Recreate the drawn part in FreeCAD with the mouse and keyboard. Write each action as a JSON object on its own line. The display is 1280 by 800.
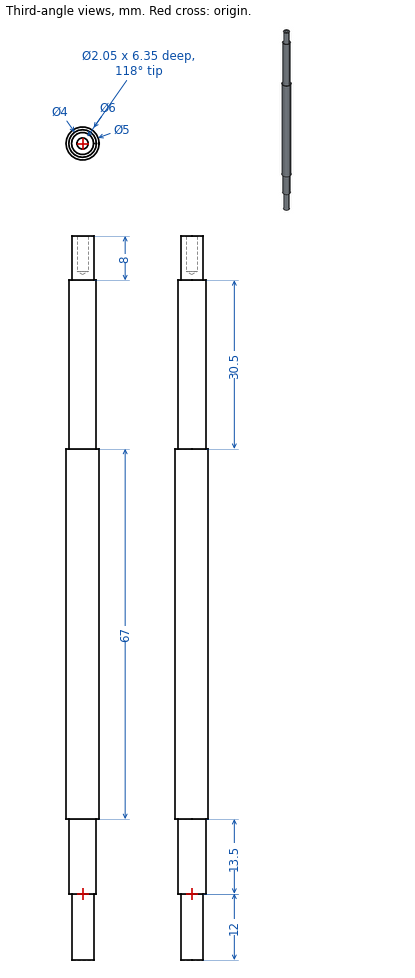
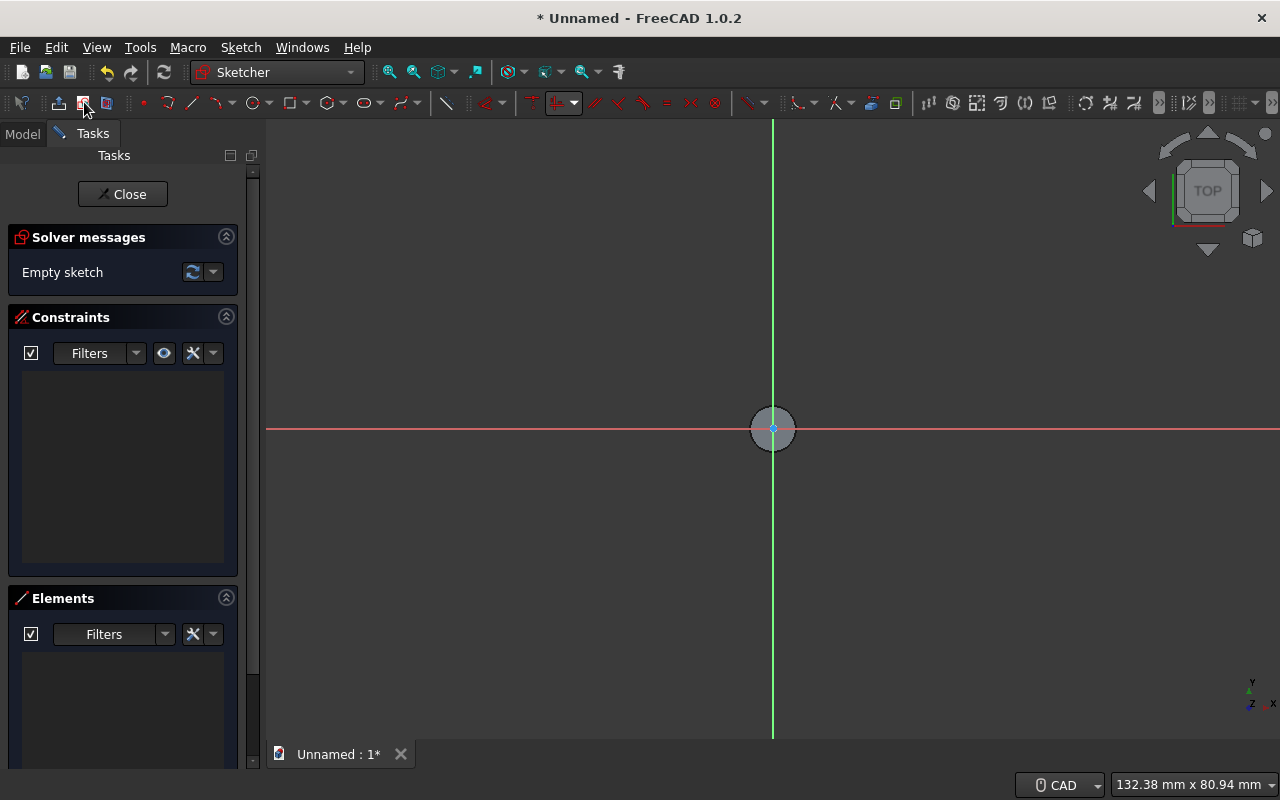
{"action": "scroll", "coordinate": [780, 429], "scroll_direction": "up", "scroll_amount": 12}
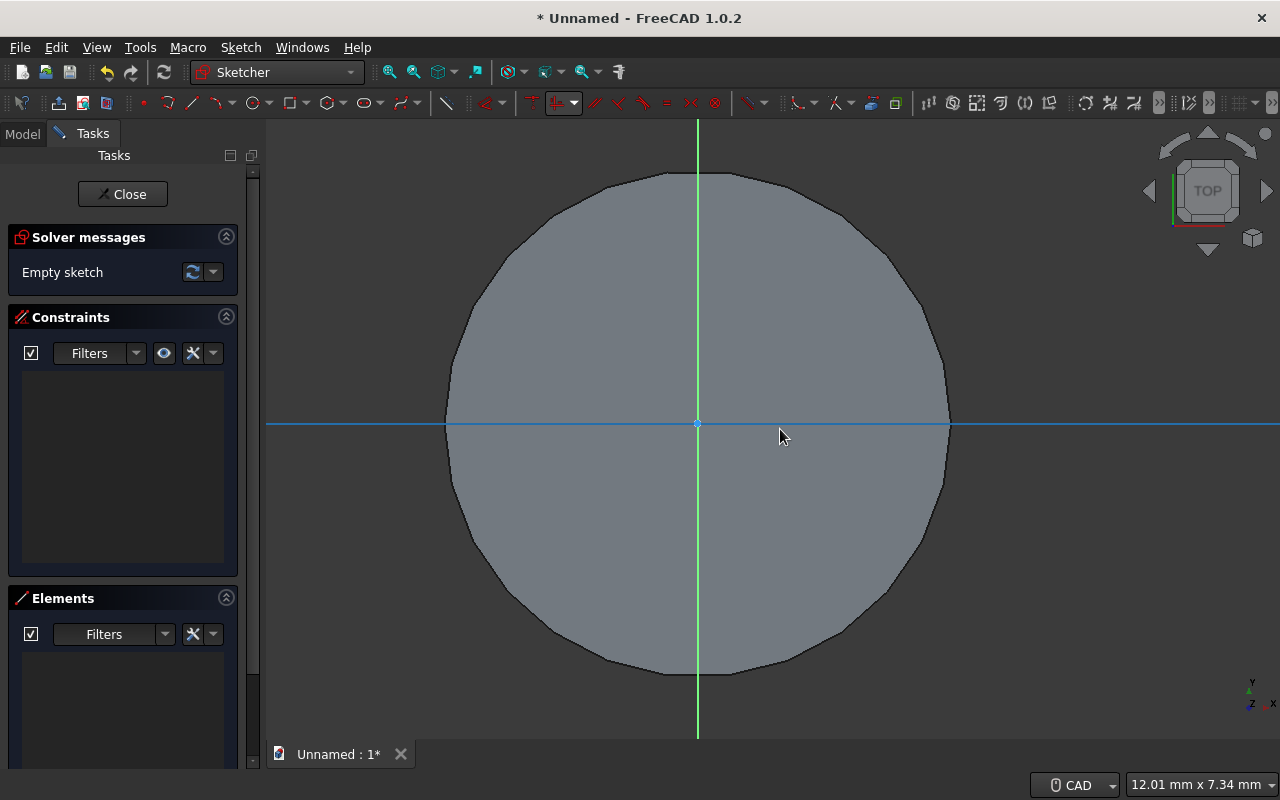
{"action": "left_click", "coordinate": [254, 104]}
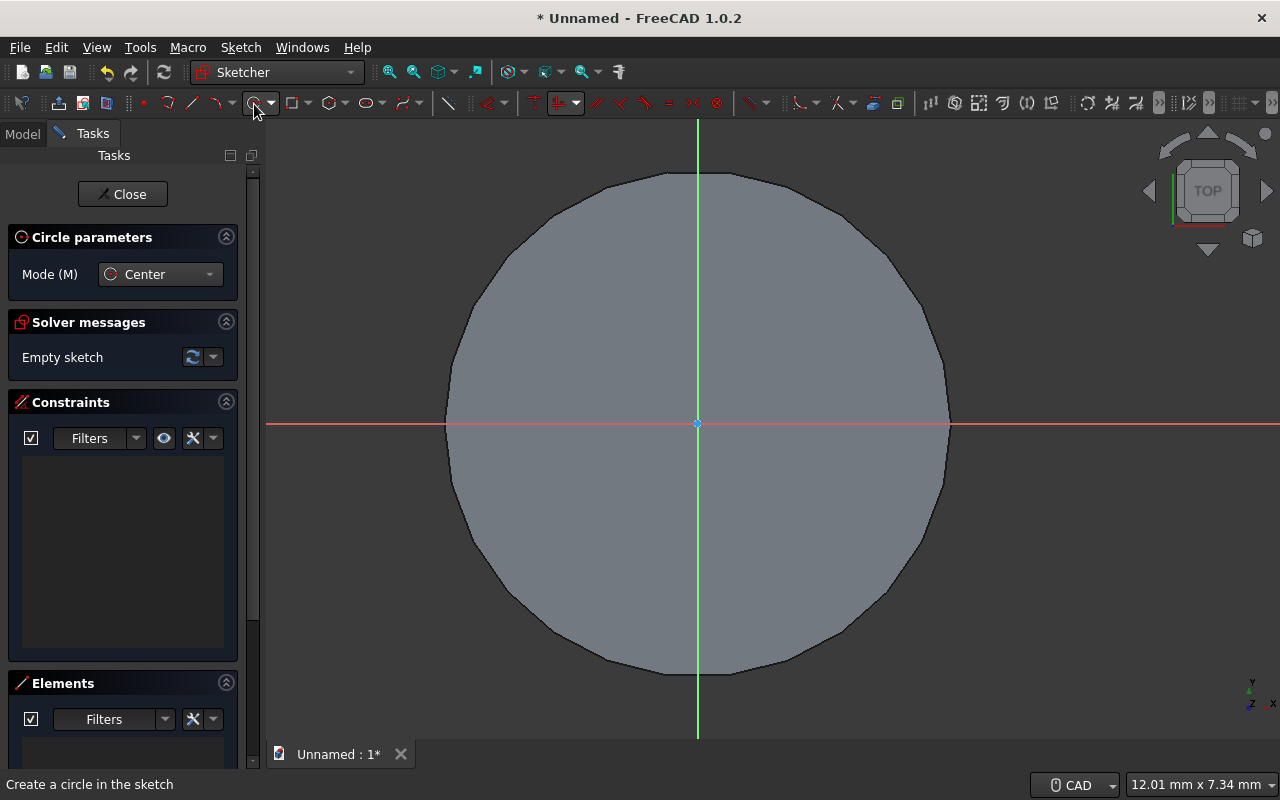
{"action": "left_click", "coordinate": [698, 424]}
{"action": "left_click", "coordinate": [847, 275]}
{"action": "key", "text": "Escape"}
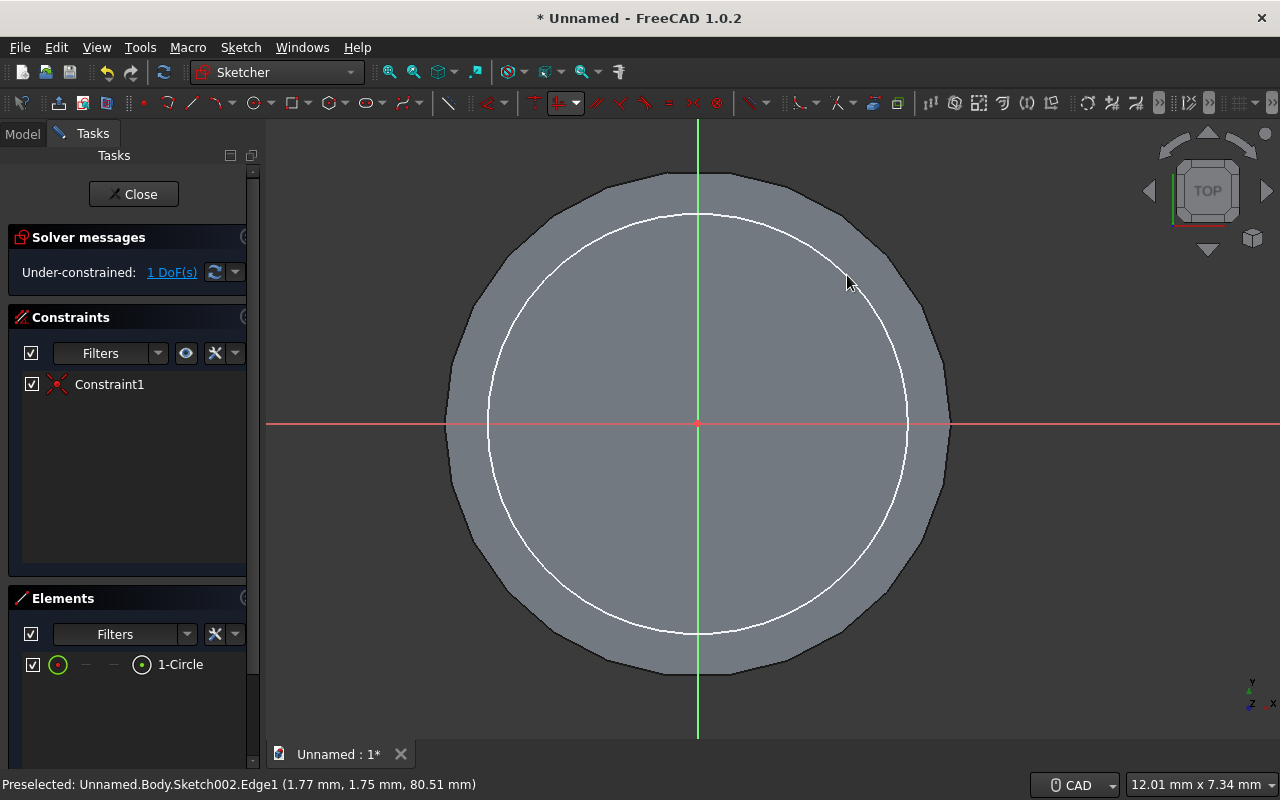
{"action": "left_click", "coordinate": [488, 104]}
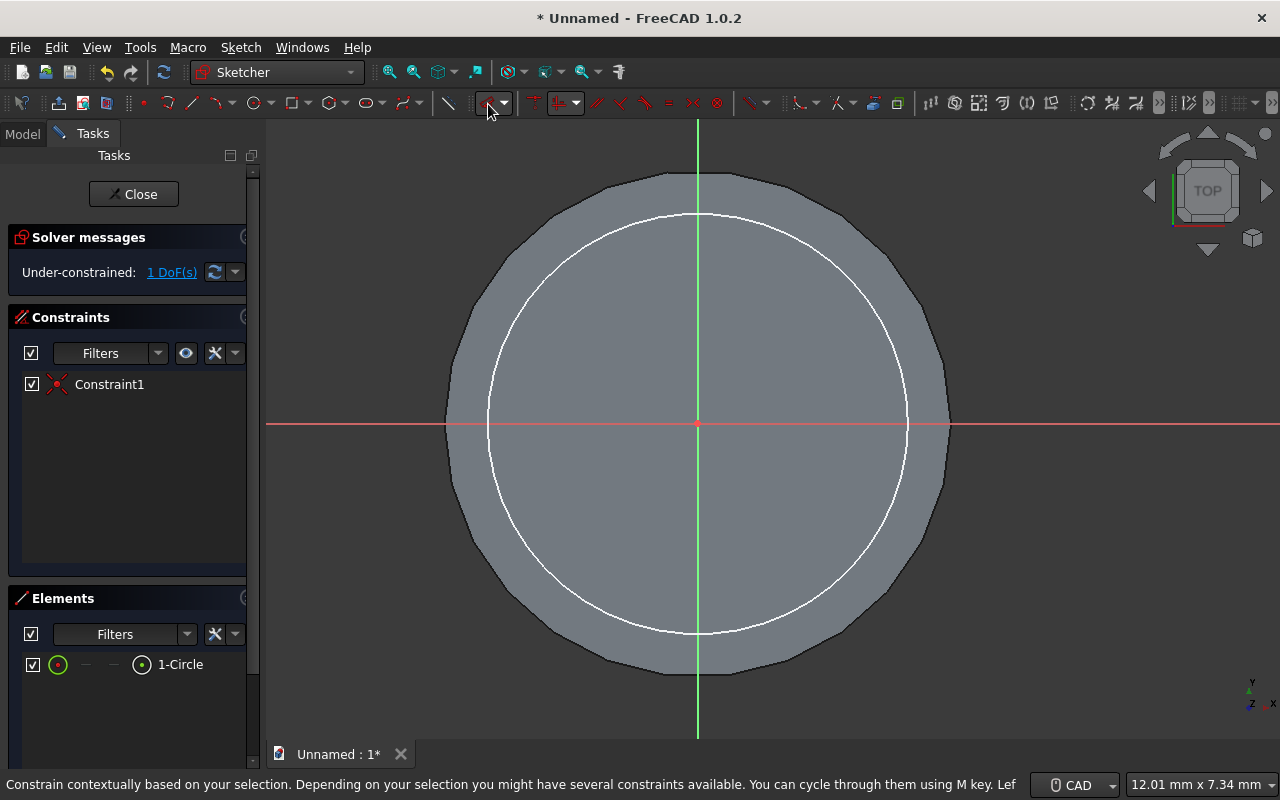
{"action": "left_click", "coordinate": [846, 275]}
{"action": "left_click", "coordinate": [869, 252]}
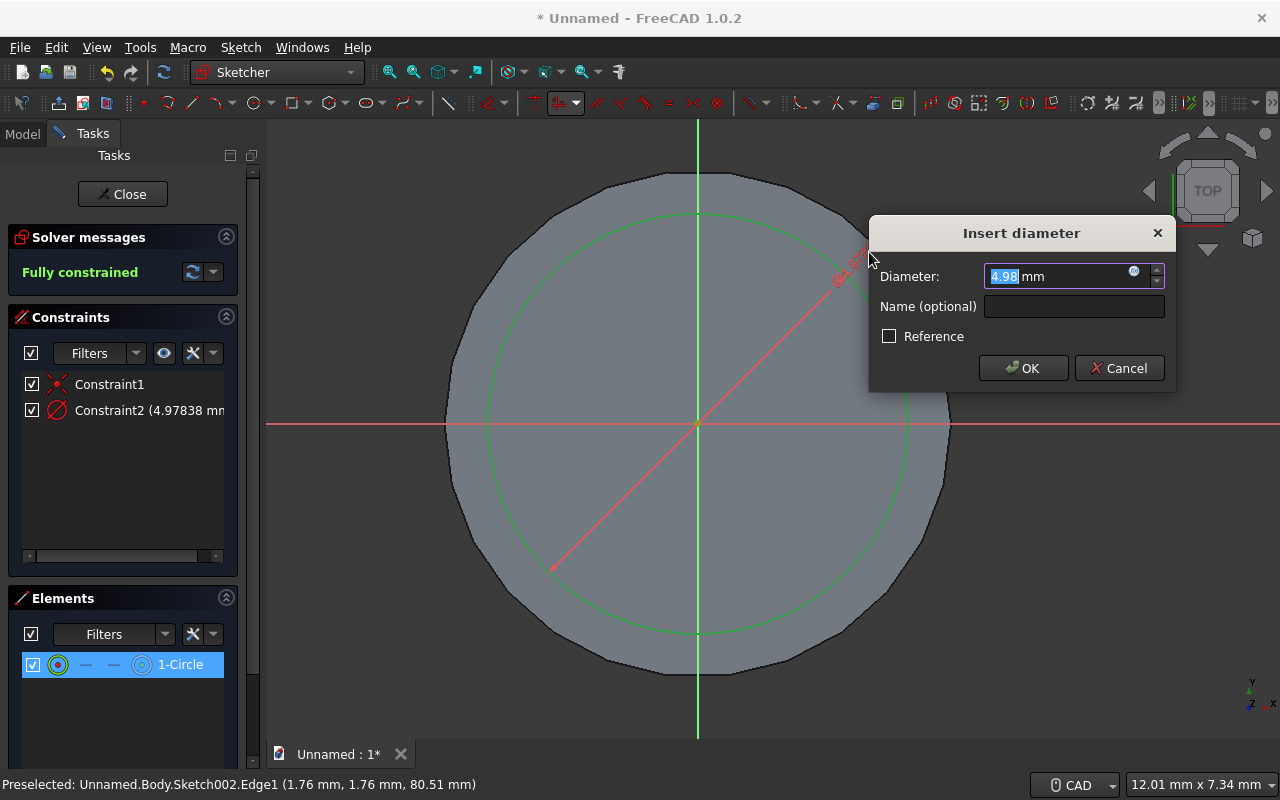
{"action": "type", "text": "5"}
{"action": "key", "text": "Return"}
{"action": "key", "text": "Escape"}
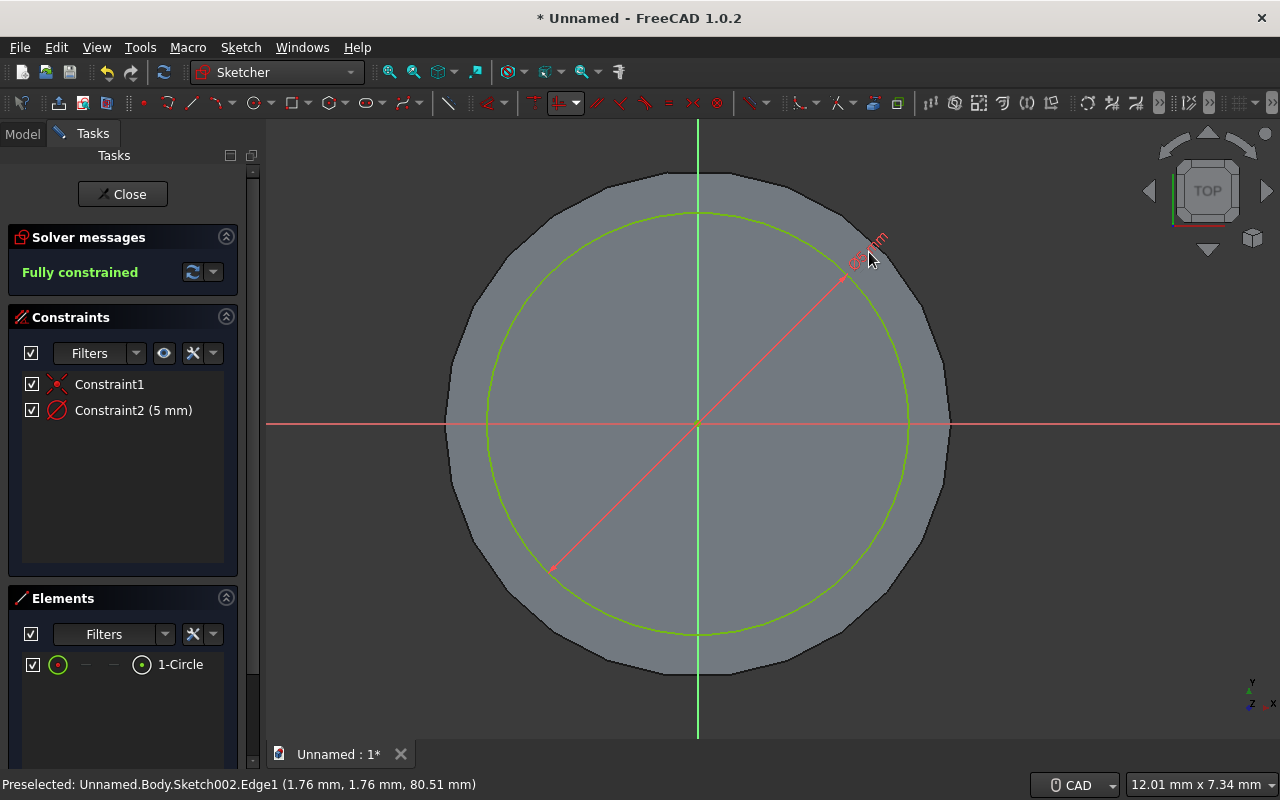
{"action": "left_click", "coordinate": [123, 194]}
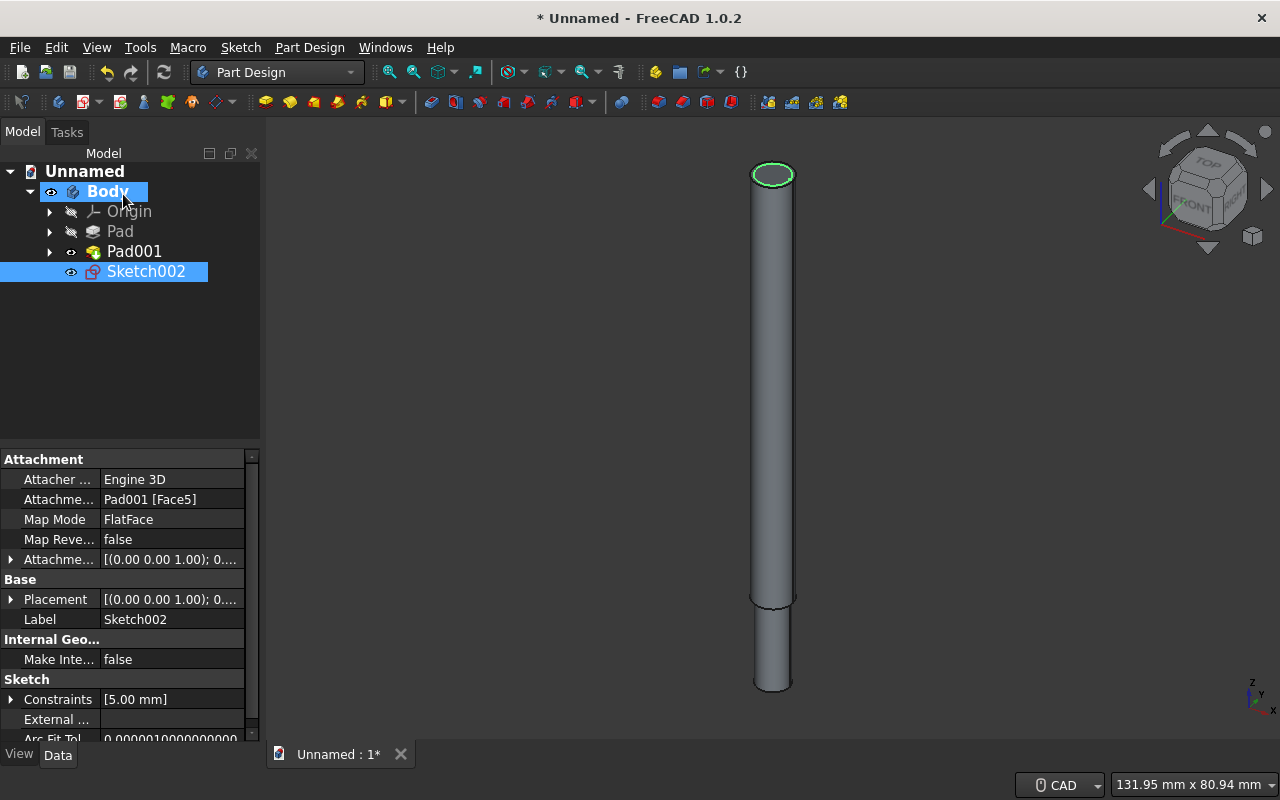
{"action": "left_click", "coordinate": [266, 102]}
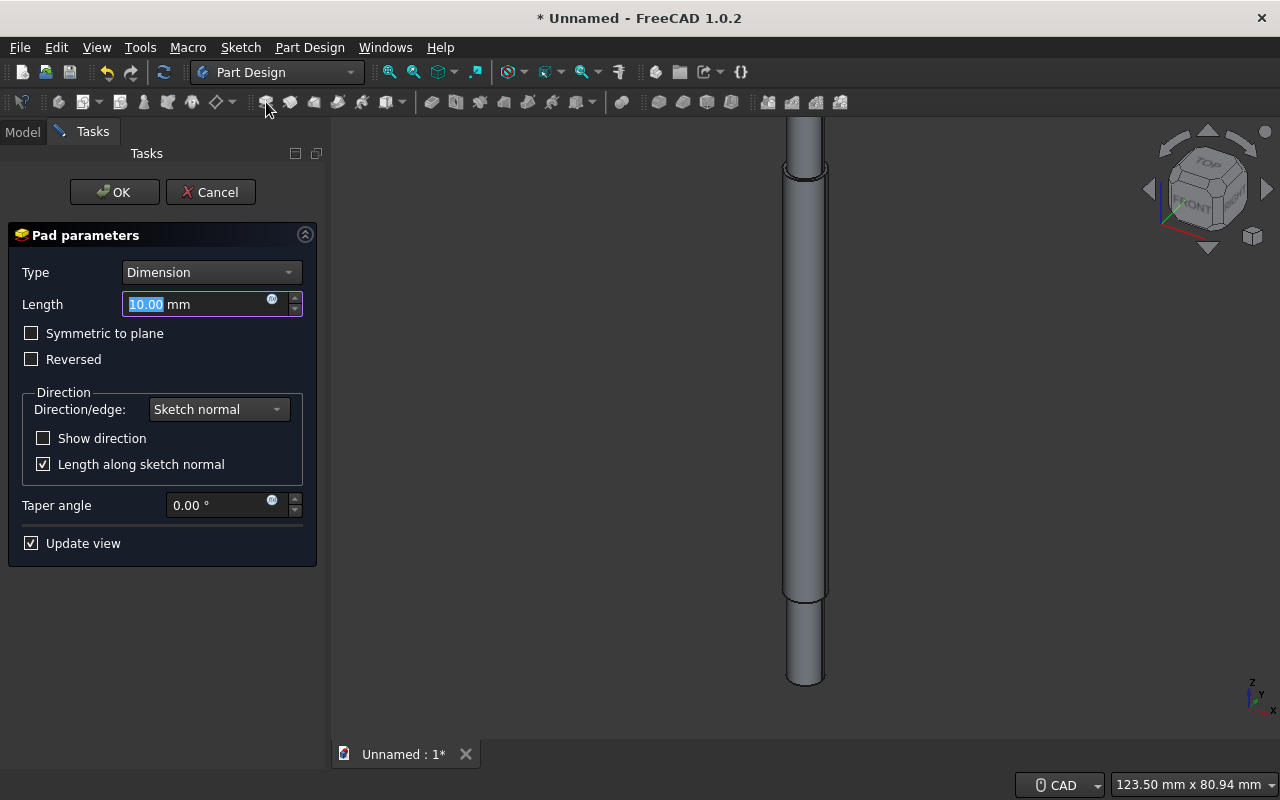
{"action": "type", "text": "30.5"}
{"action": "key", "text": "Tab"}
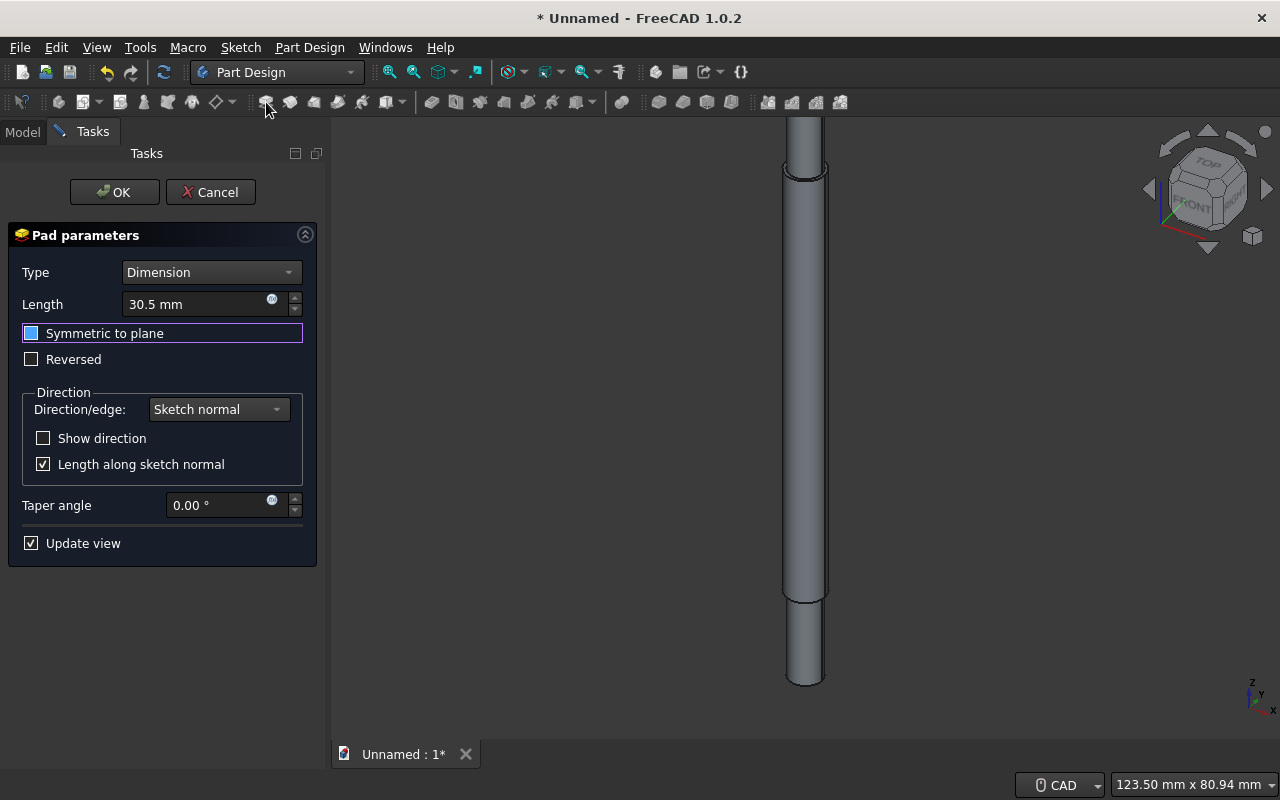
{"action": "left_click", "coordinate": [115, 192]}